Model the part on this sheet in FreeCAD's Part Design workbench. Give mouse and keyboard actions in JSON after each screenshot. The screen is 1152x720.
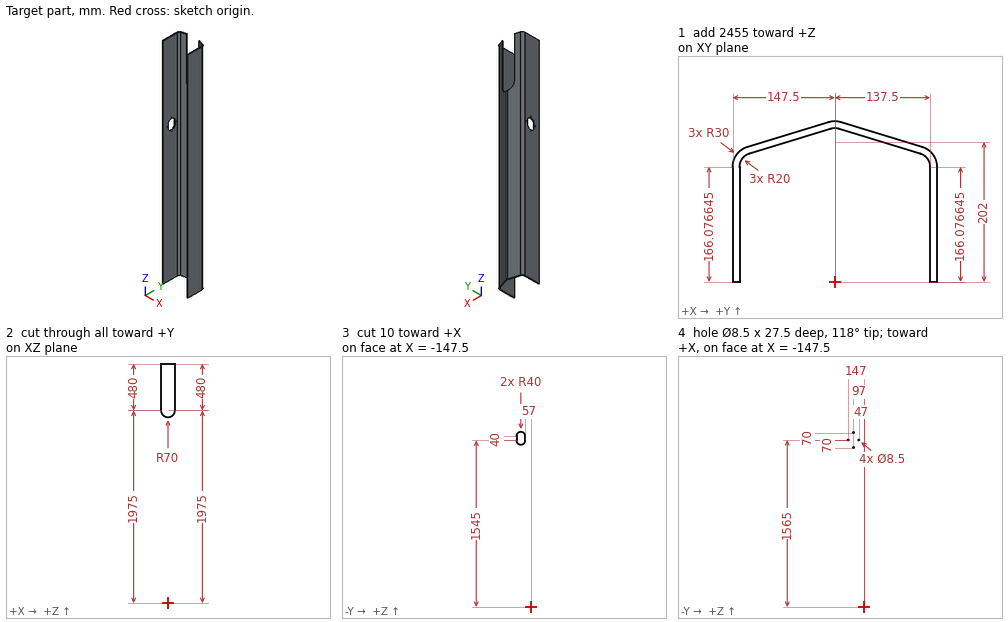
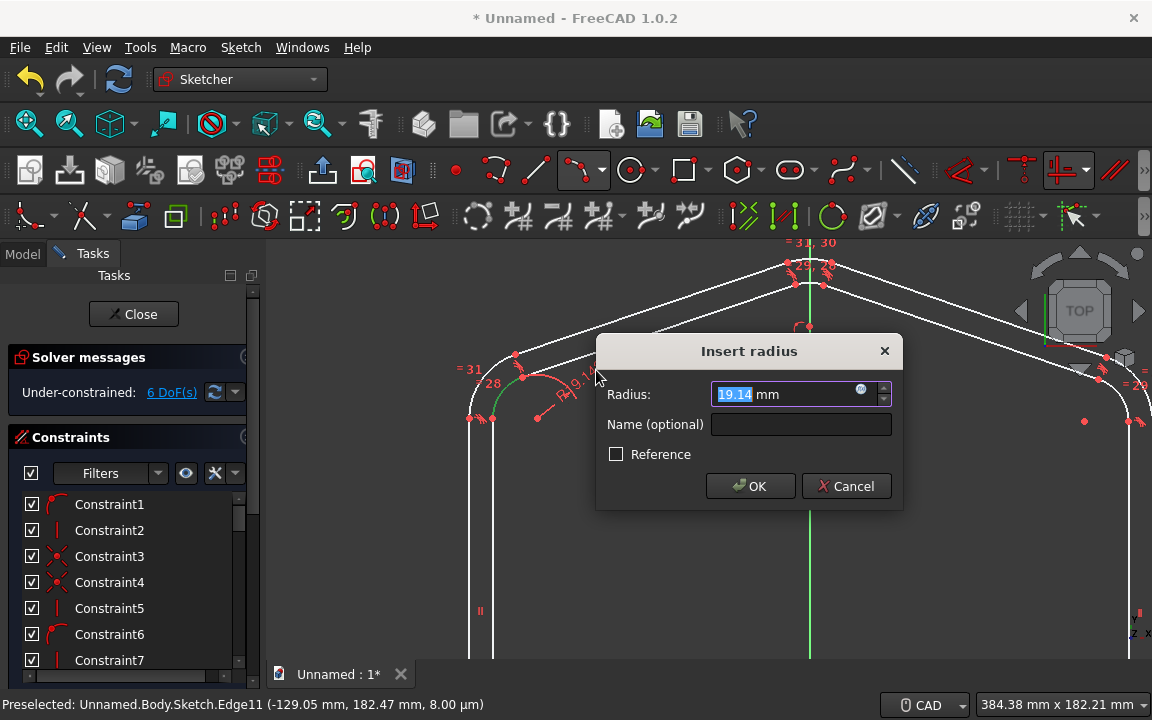
{"action": "type", "text": "20"}
{"action": "key", "text": "Return"}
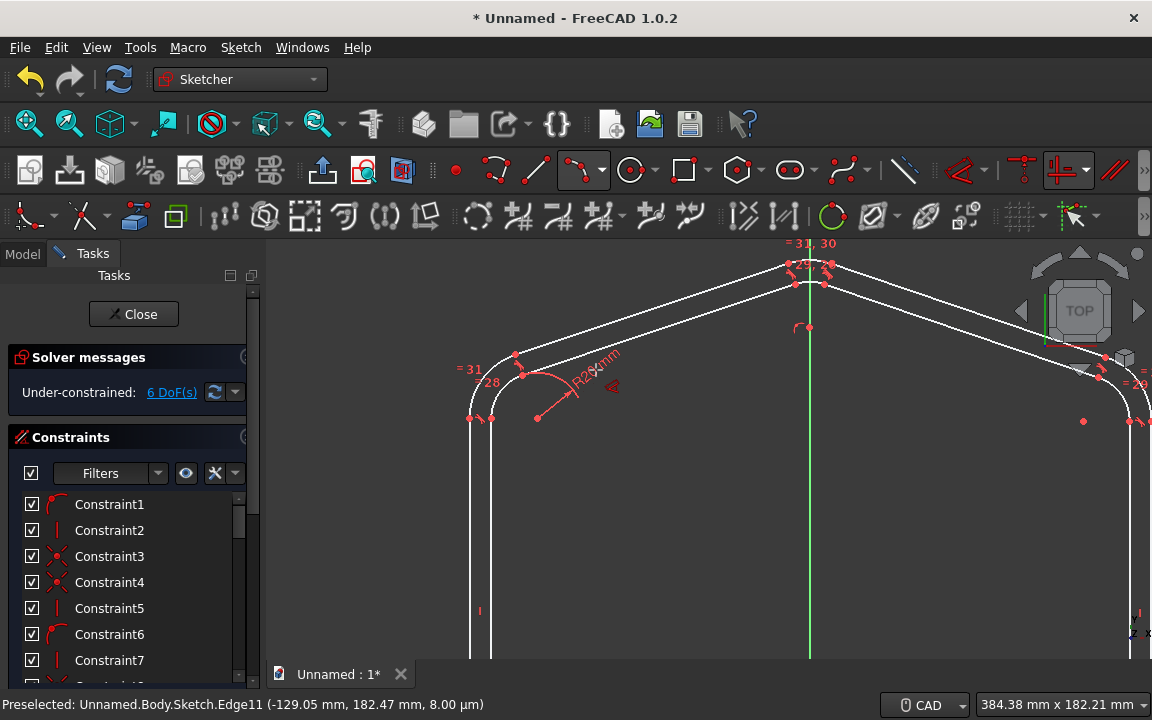
{"action": "scroll", "coordinate": [503, 378], "scroll_direction": "down", "scroll_amount": 4}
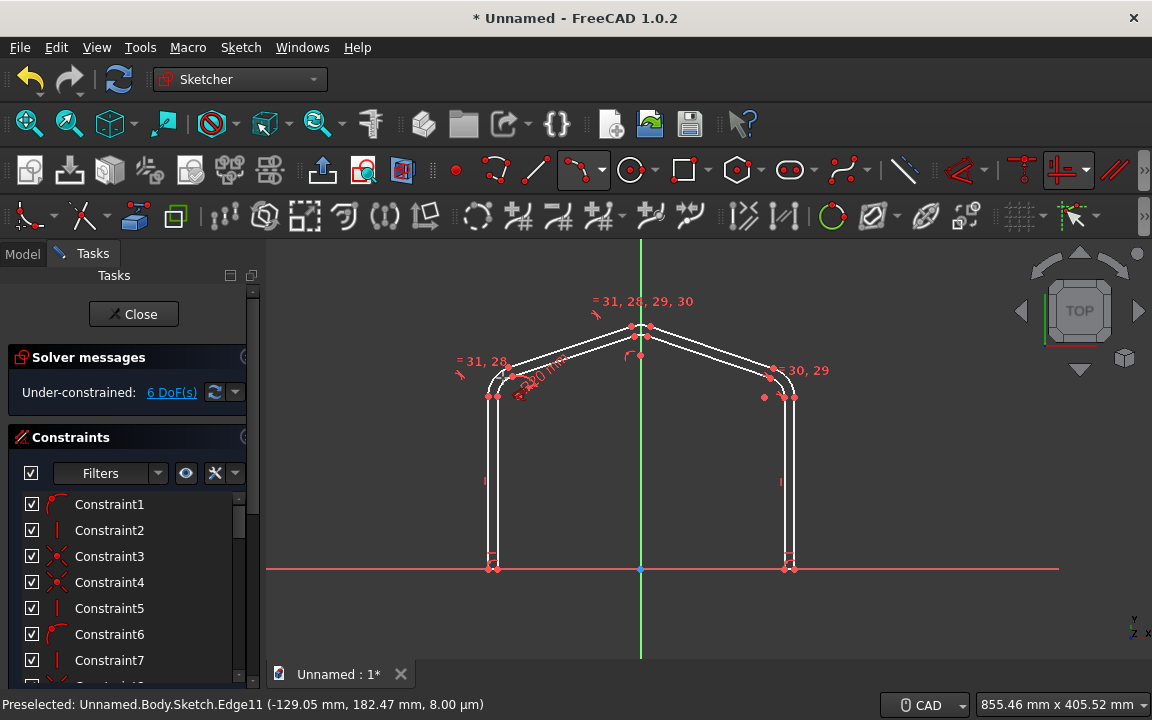
{"action": "scroll", "coordinate": [792, 387], "scroll_direction": "up", "scroll_amount": 2}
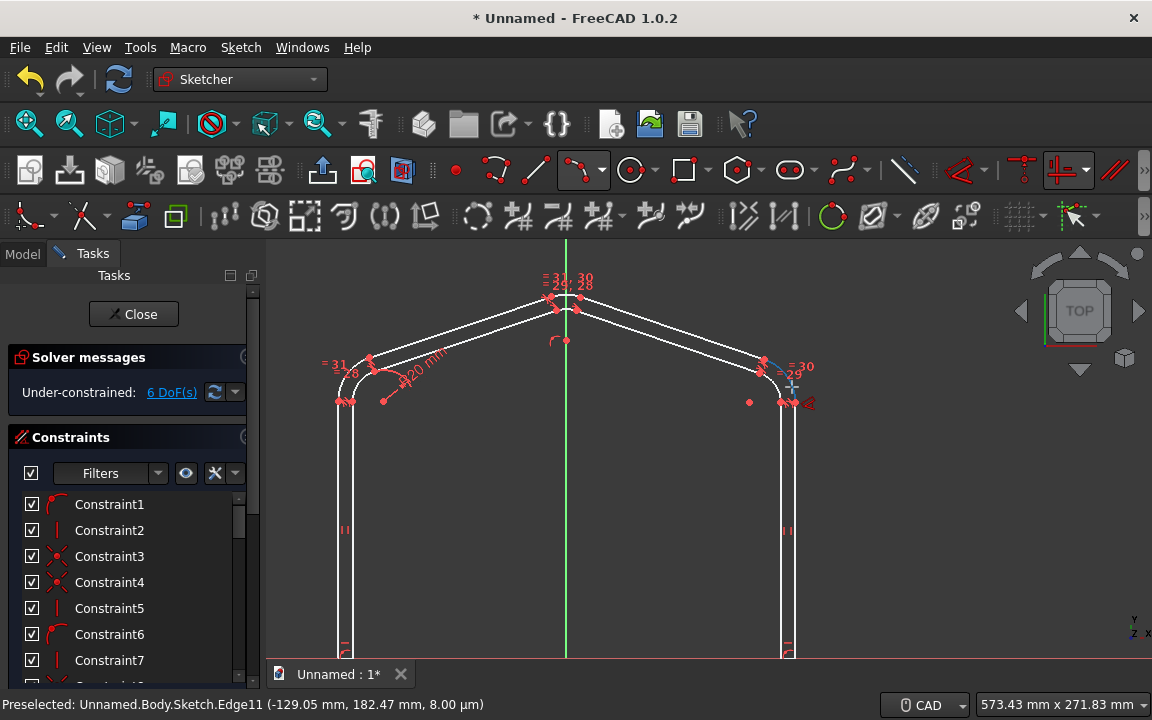
{"action": "left_click", "coordinate": [792, 386]}
{"action": "left_click", "coordinate": [822, 374]}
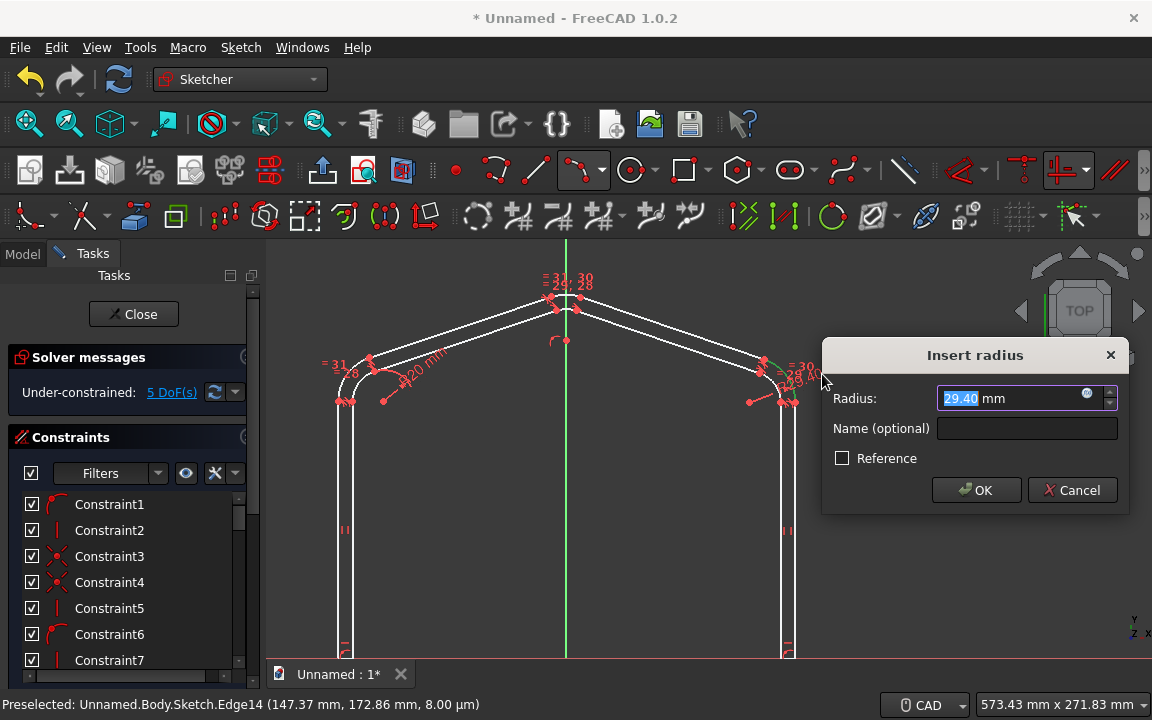
{"action": "type", "text": "30"}
{"action": "key", "text": "Return"}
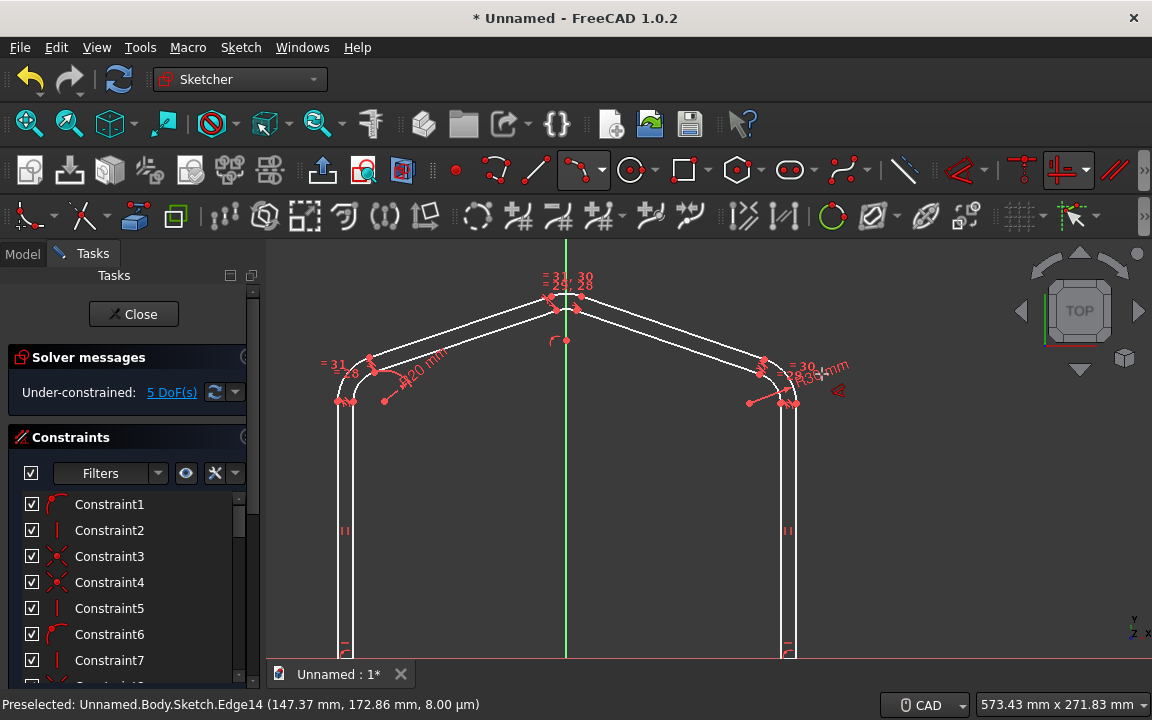
{"action": "left_click", "coordinate": [566, 340]}
{"action": "left_click", "coordinate": [600, 486]}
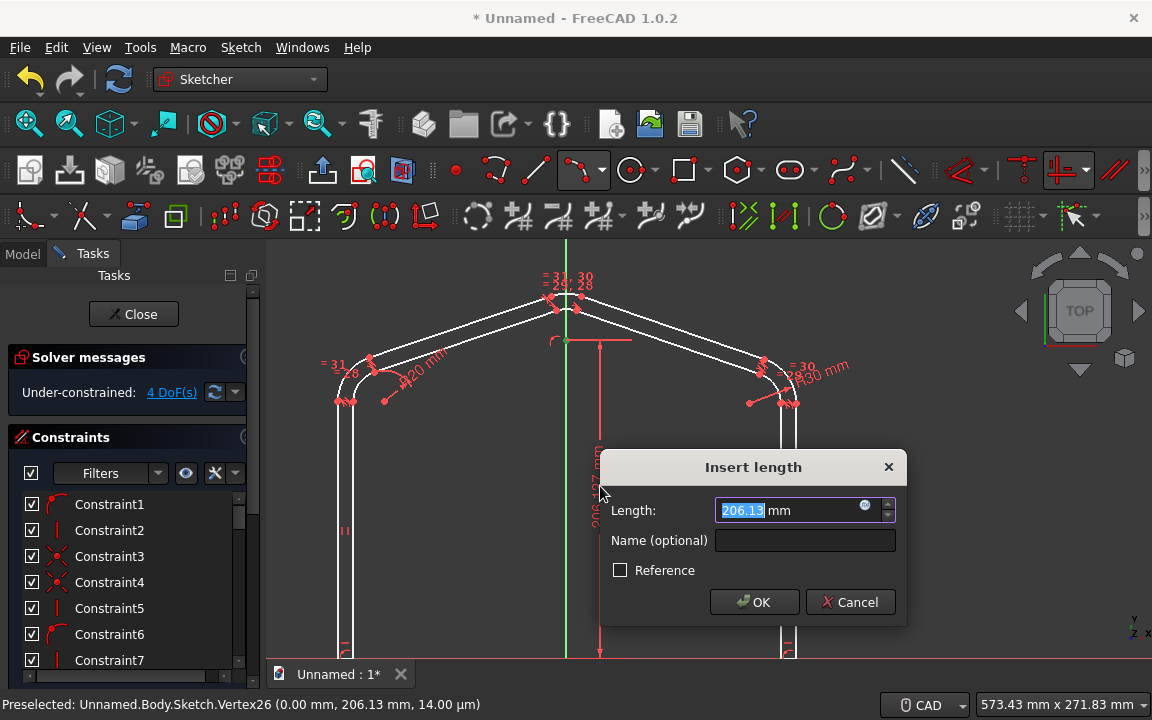
{"action": "type", "text": "202"}
{"action": "key", "text": "Return"}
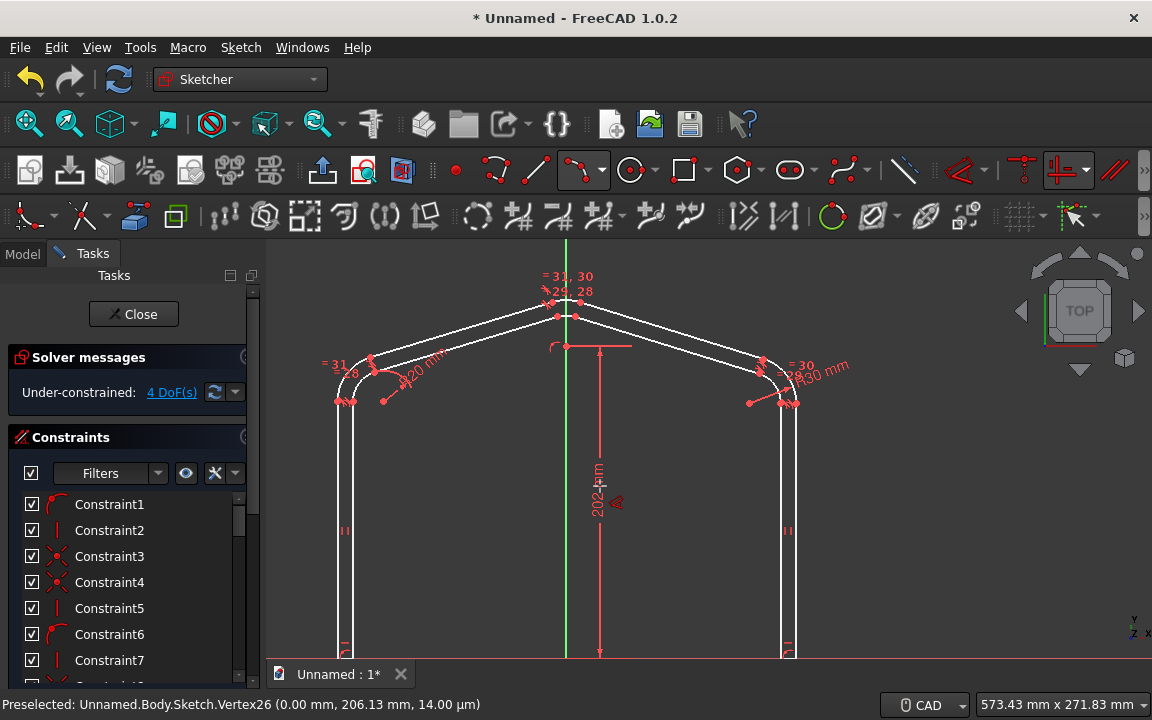
{"action": "left_click", "coordinate": [338, 402]}
{"action": "left_click", "coordinate": [505, 368]}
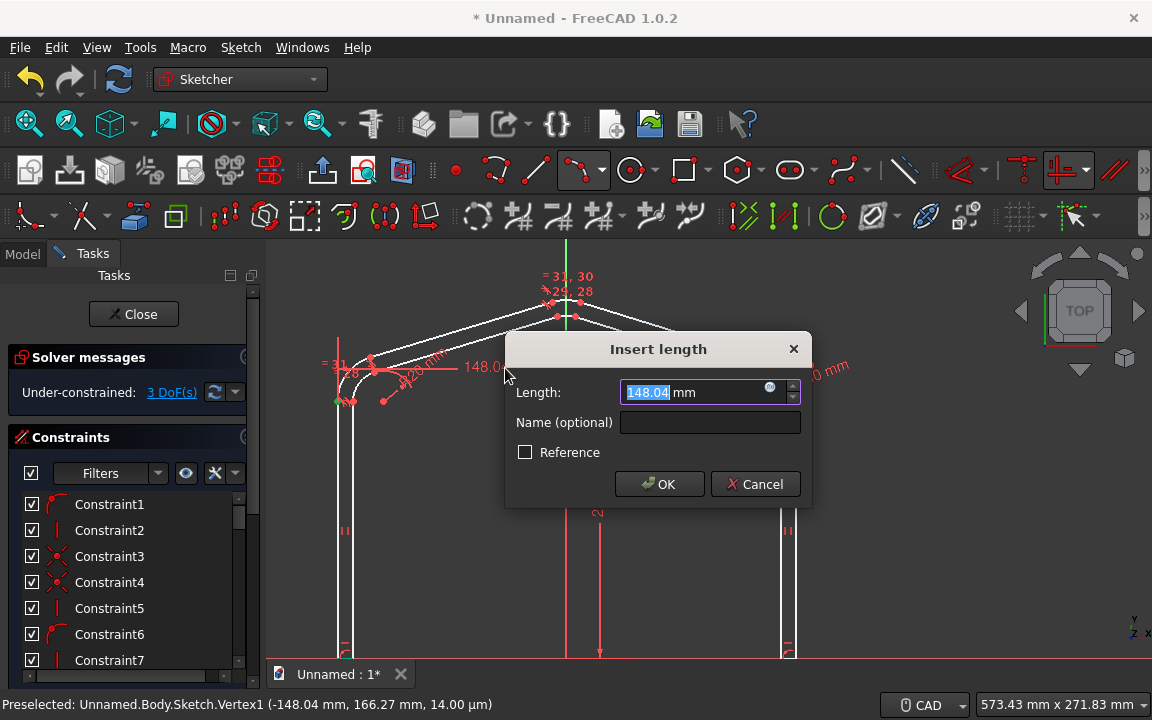
{"action": "type", "text": "147.5"}
{"action": "key", "text": "Return"}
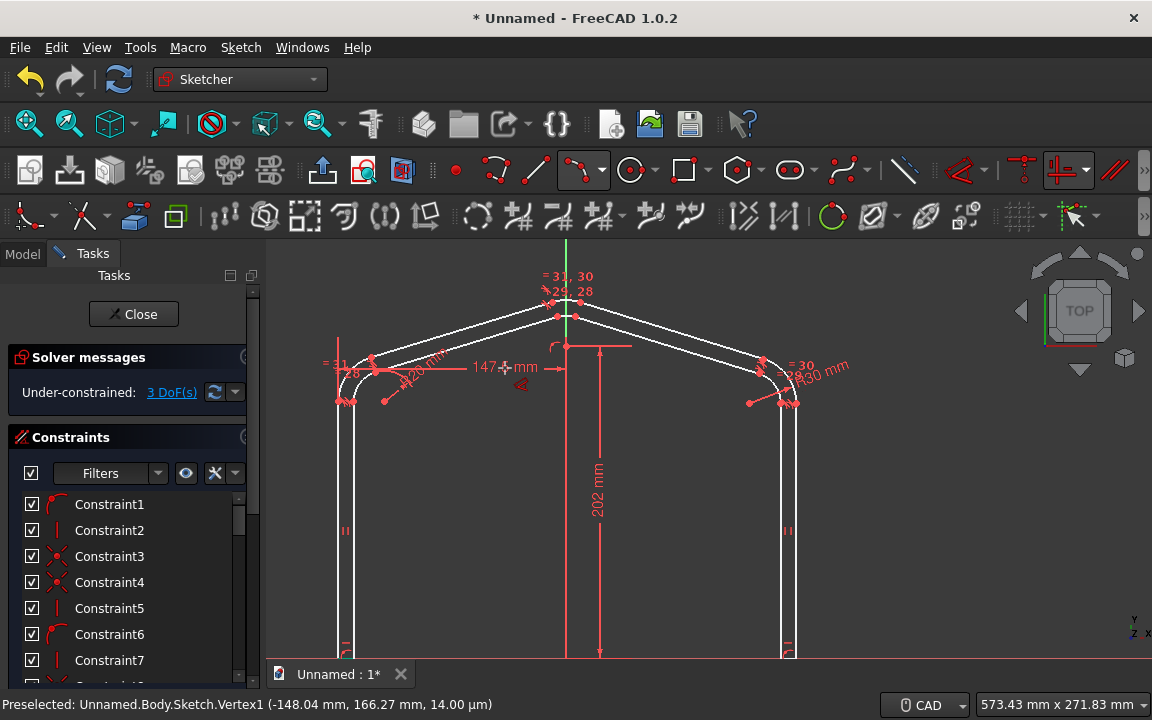
{"action": "left_click", "coordinate": [781, 403]}
{"action": "left_click", "coordinate": [674, 369]}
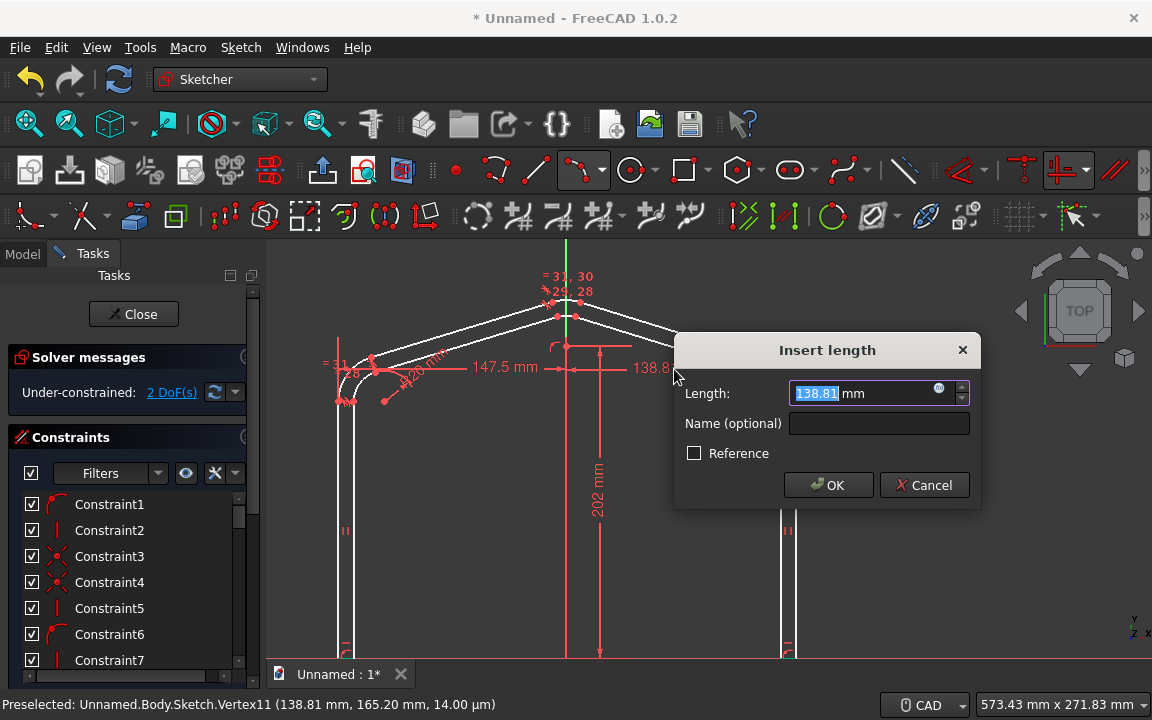
{"action": "type", "text": "137.5"}
{"action": "key", "text": "Return"}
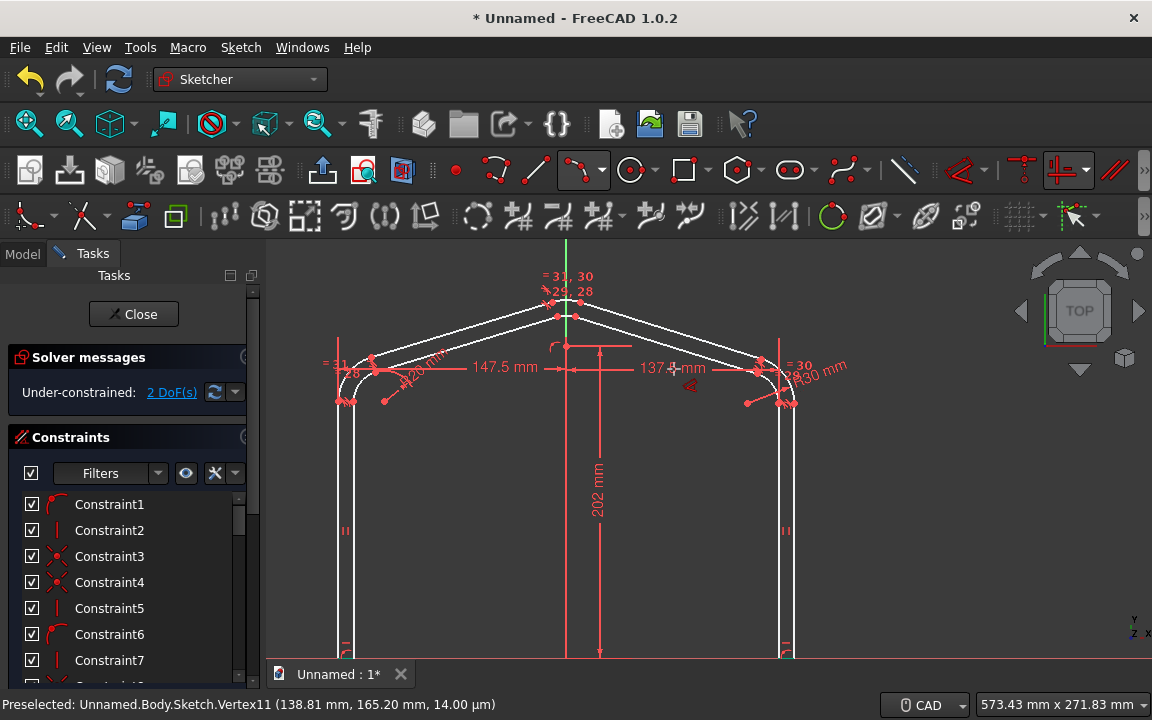
{"action": "left_click", "coordinate": [338, 479]}
{"action": "left_click", "coordinate": [304, 516]}